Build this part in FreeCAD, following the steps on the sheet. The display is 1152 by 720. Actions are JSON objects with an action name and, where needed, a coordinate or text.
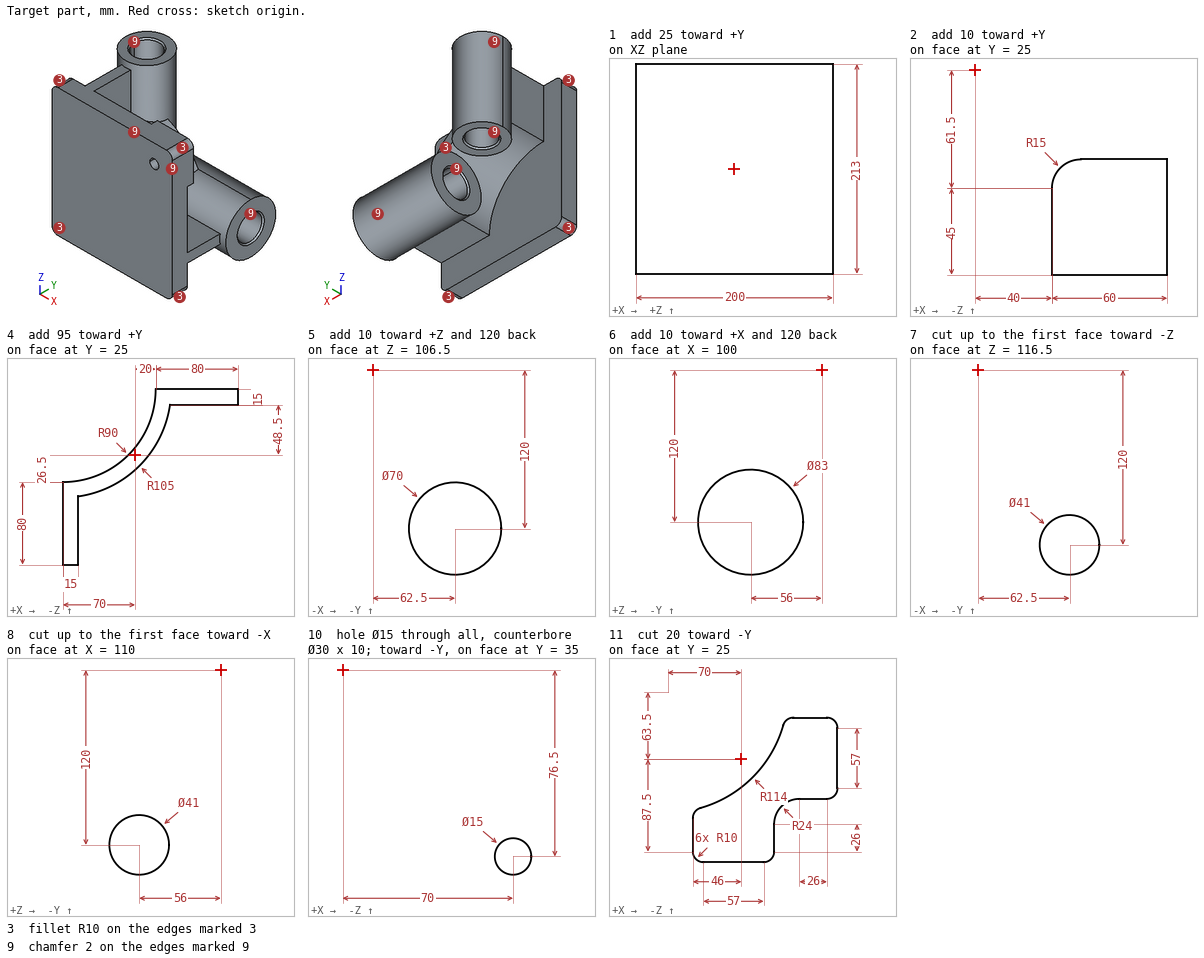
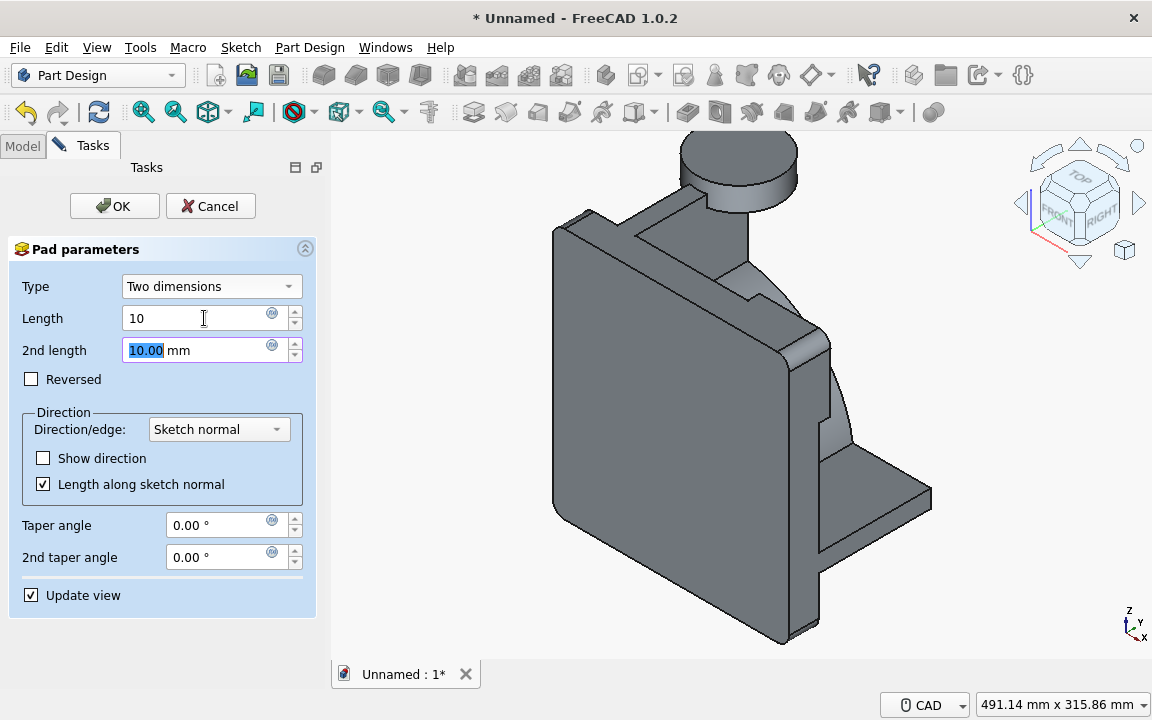
{"action": "type", "text": "120"}
{"action": "key", "text": "Tab"}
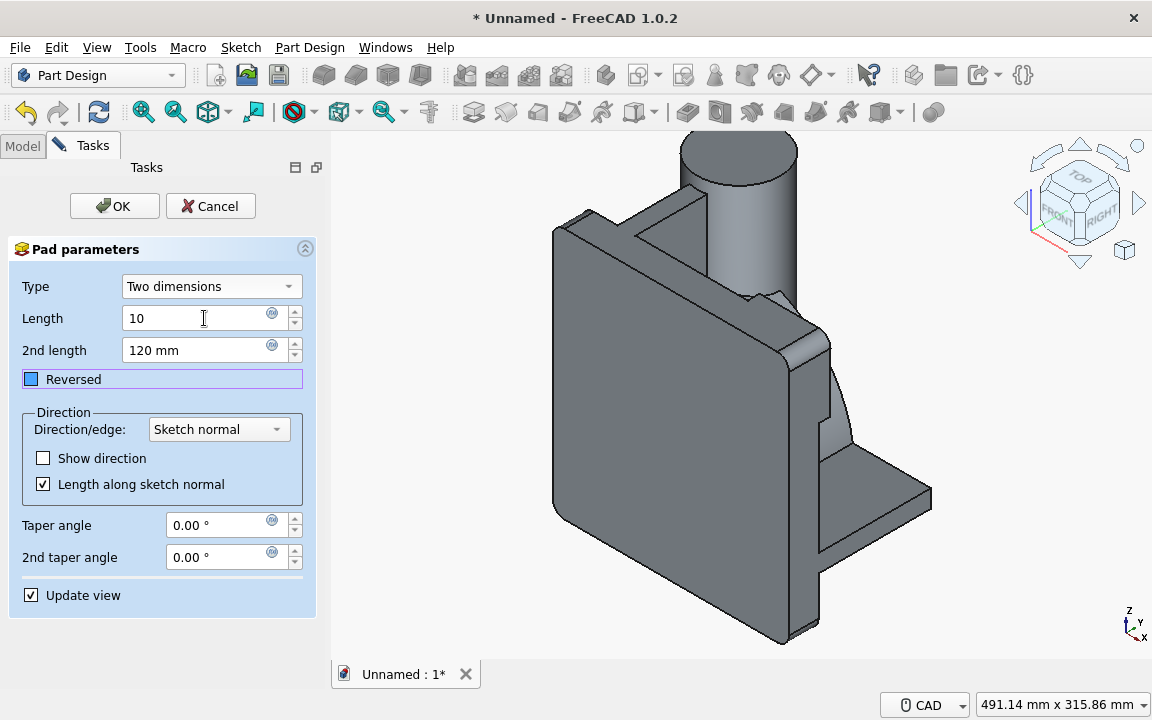
{"action": "left_click", "coordinate": [115, 206]}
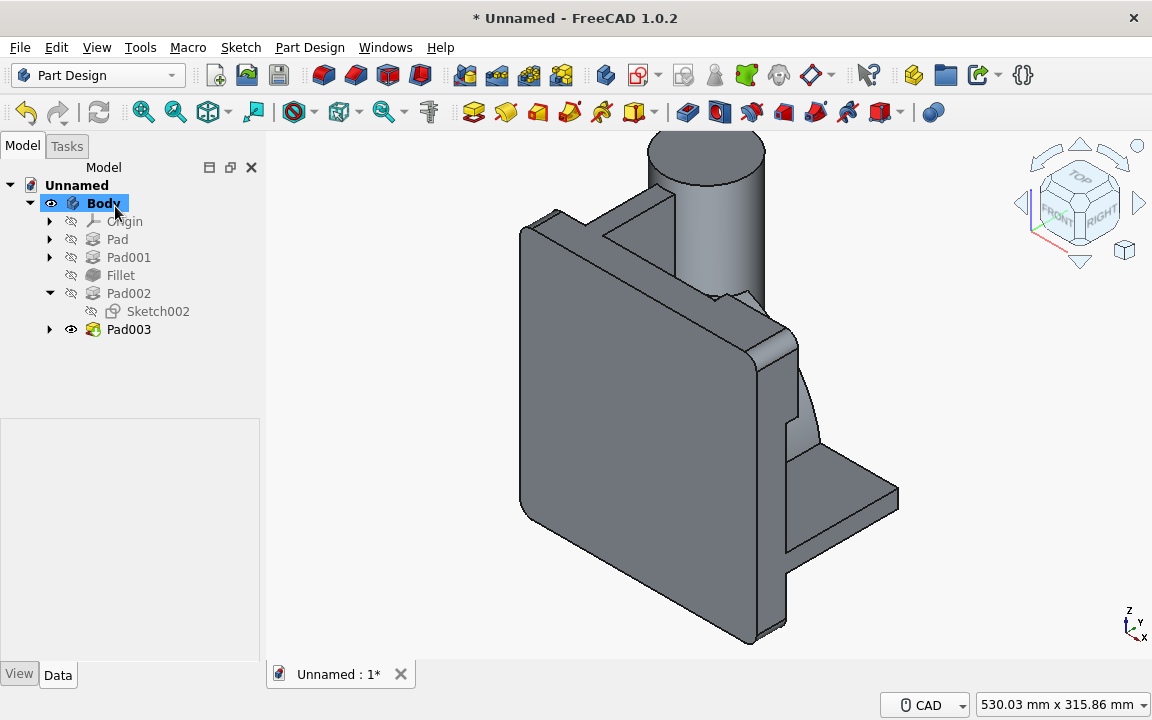
{"action": "left_click", "coordinate": [144, 112]}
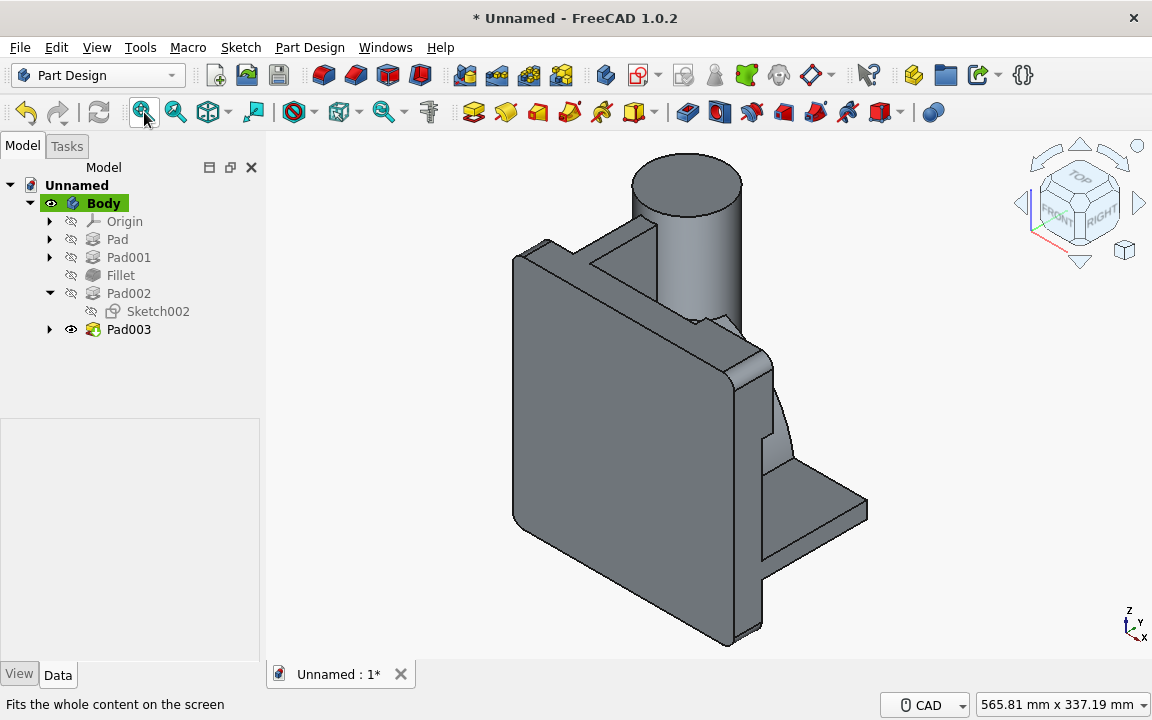
{"action": "left_click", "coordinate": [762, 392]}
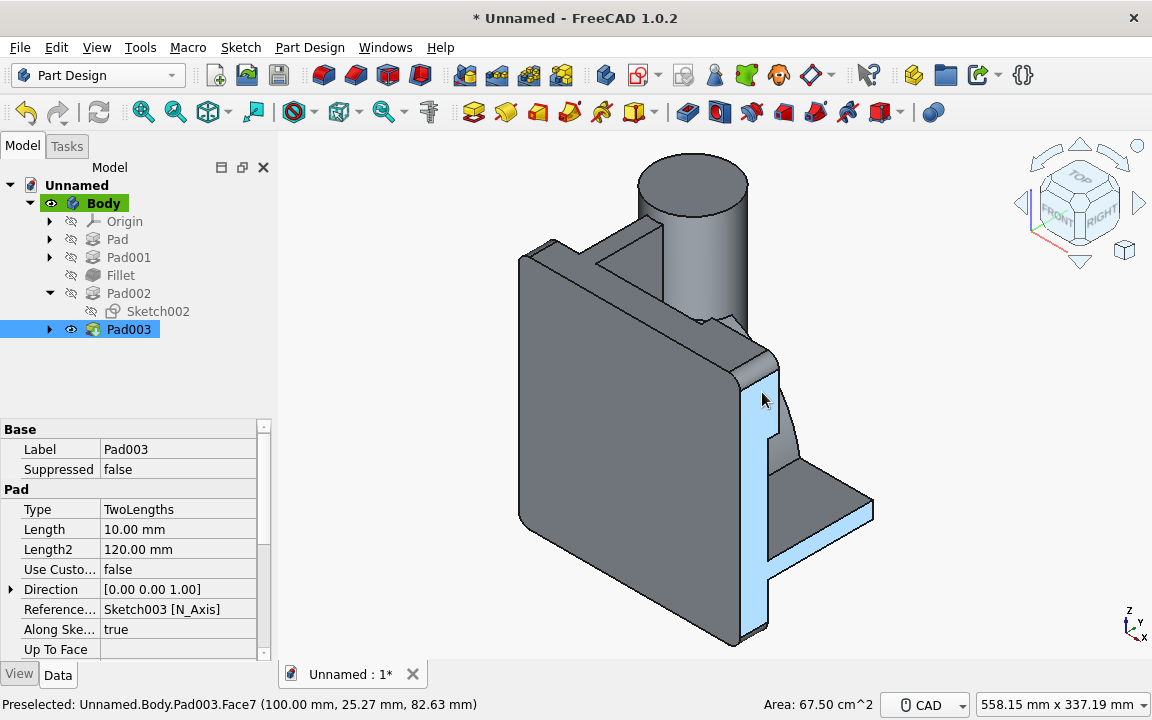
{"action": "left_click", "coordinate": [638, 76]}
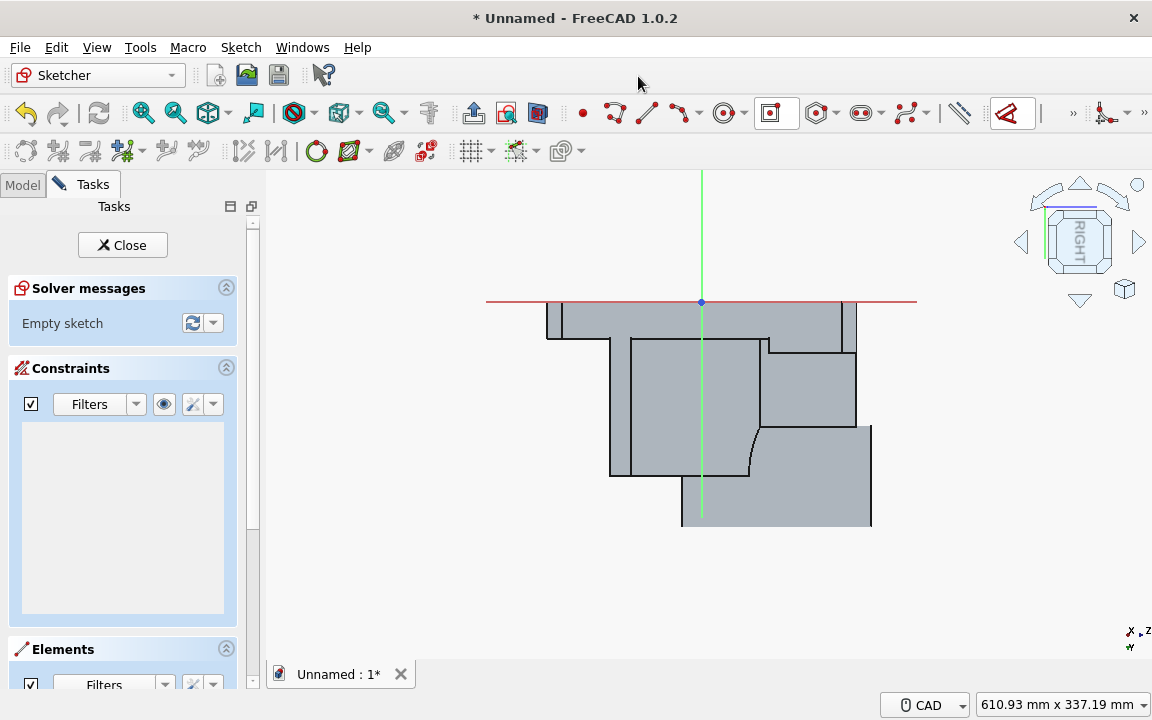
{"action": "left_click", "coordinate": [724, 114]}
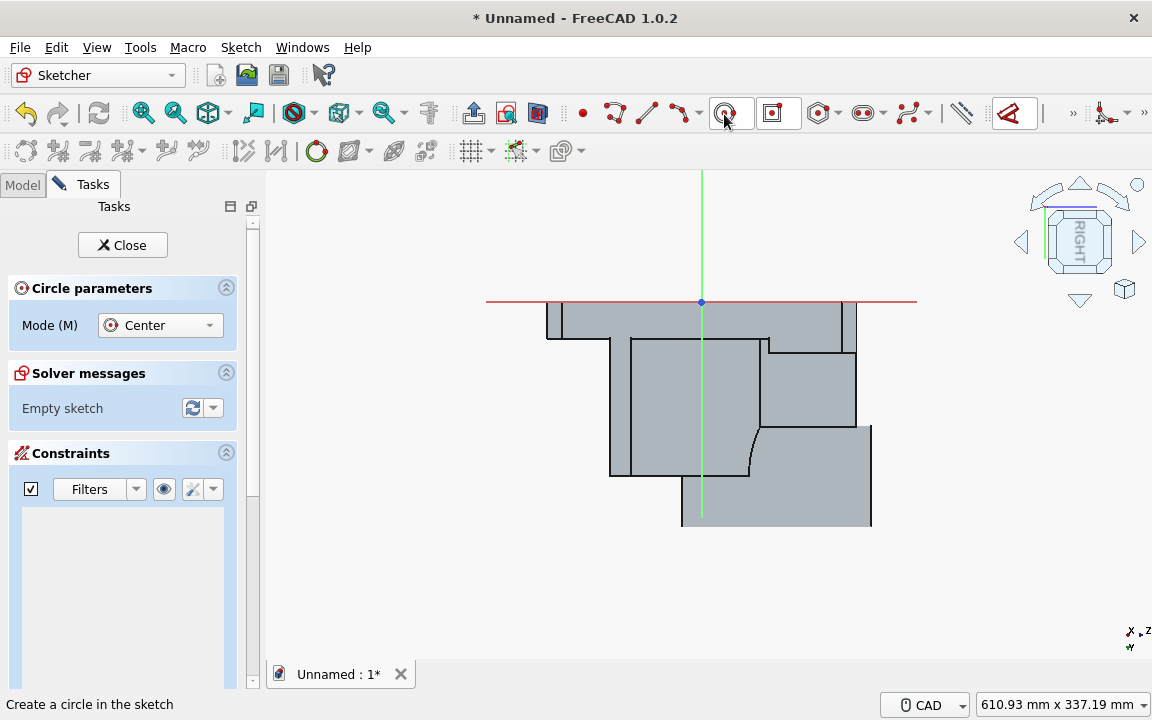
{"action": "left_click", "coordinate": [621, 476]}
{"action": "mouse_move", "coordinate": [663, 434]}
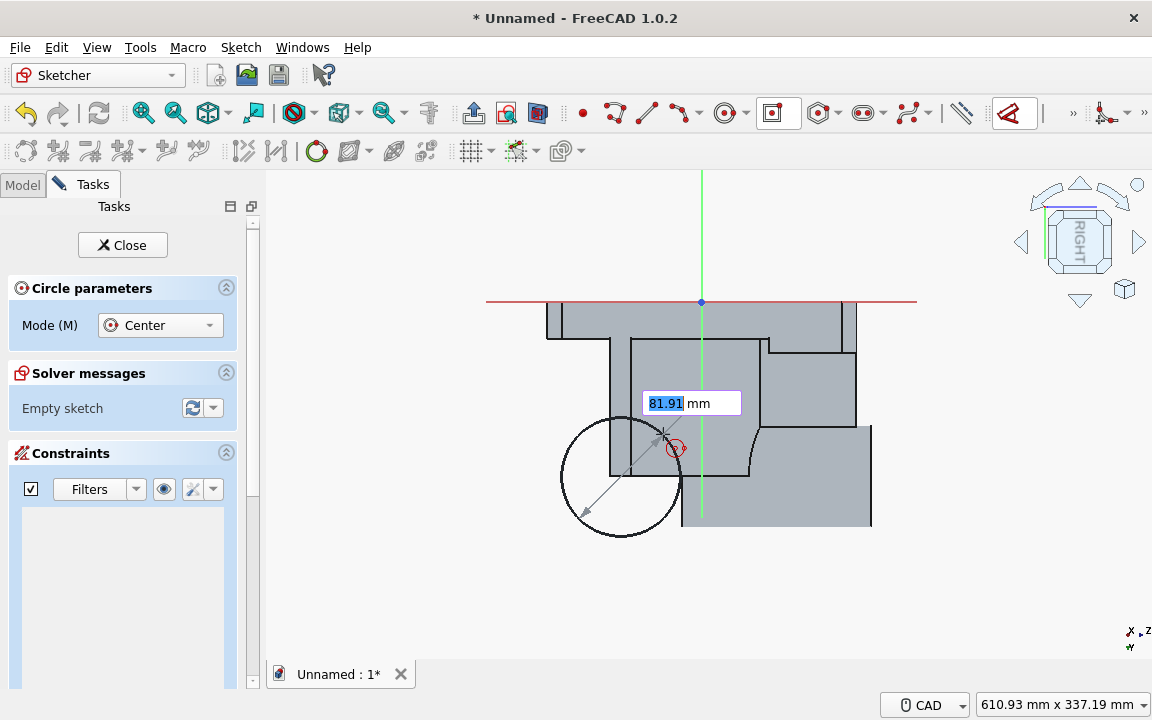
{"action": "type", "text": "83"}
{"action": "key", "text": "Return"}
{"action": "key", "text": "Escape"}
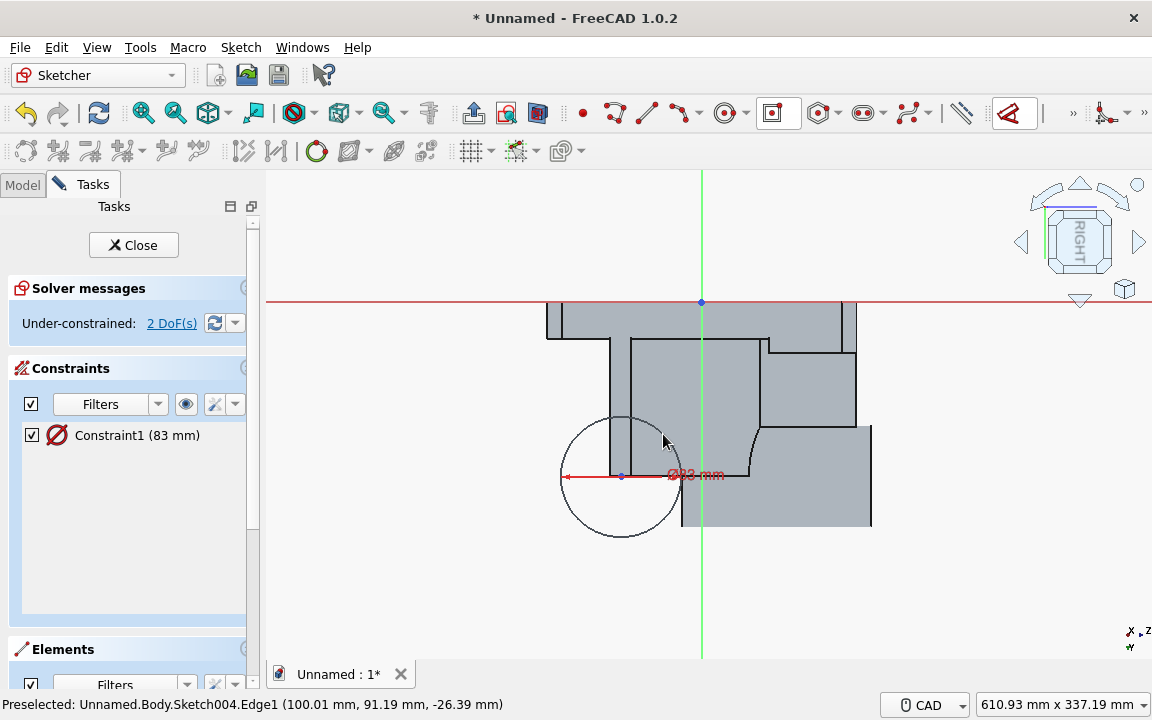
{"action": "left_click", "coordinate": [621, 477]}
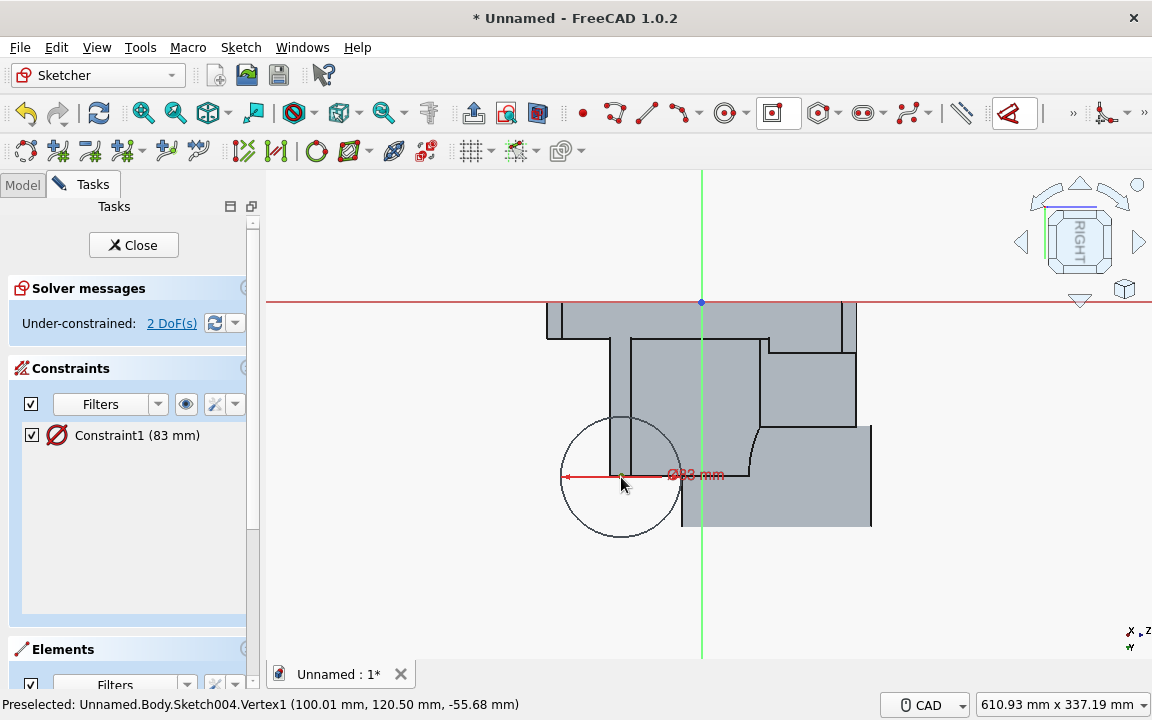
{"action": "key", "text": "l"}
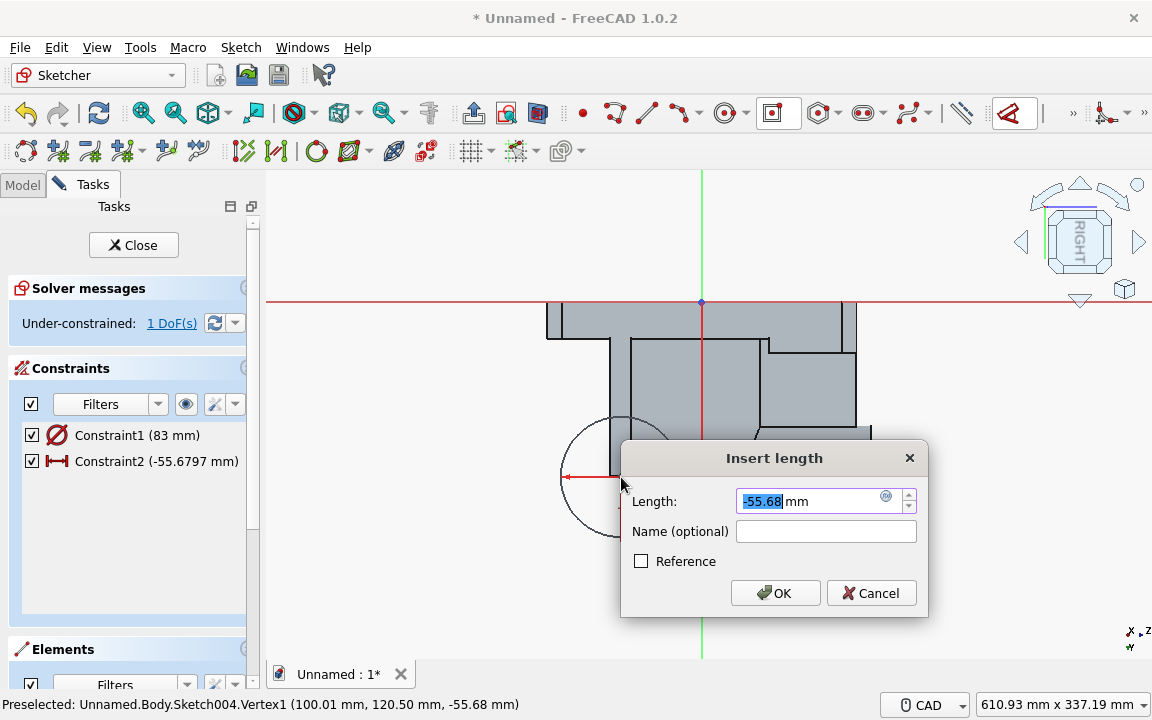
{"action": "type", "text": "-56"}
{"action": "key", "text": "Return"}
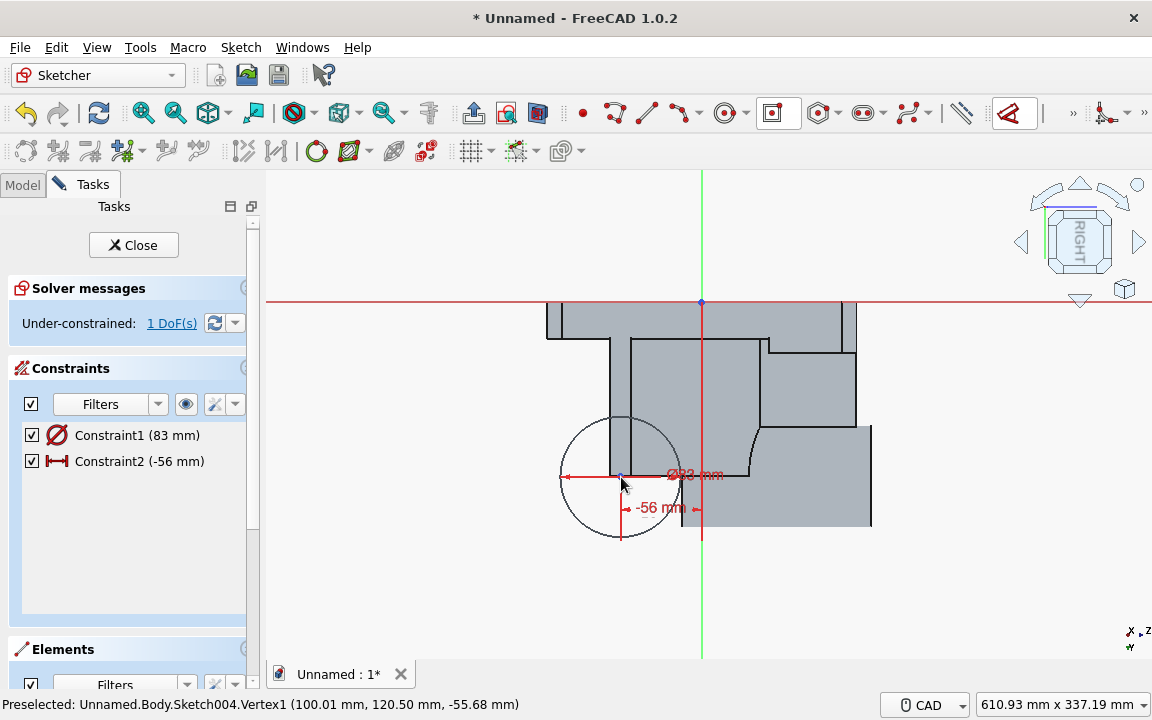
{"action": "left_click", "coordinate": [621, 477]}